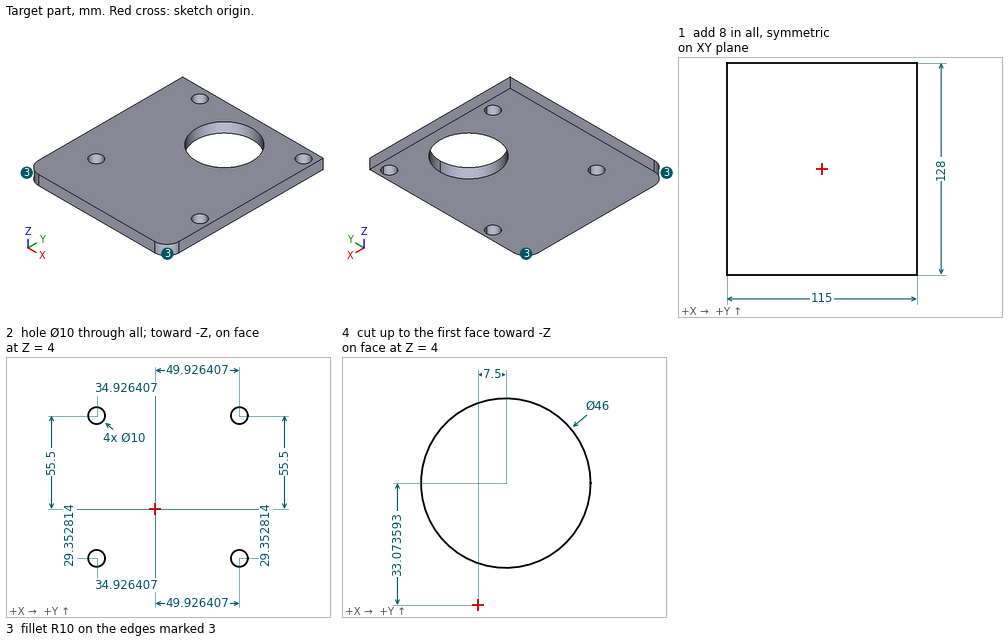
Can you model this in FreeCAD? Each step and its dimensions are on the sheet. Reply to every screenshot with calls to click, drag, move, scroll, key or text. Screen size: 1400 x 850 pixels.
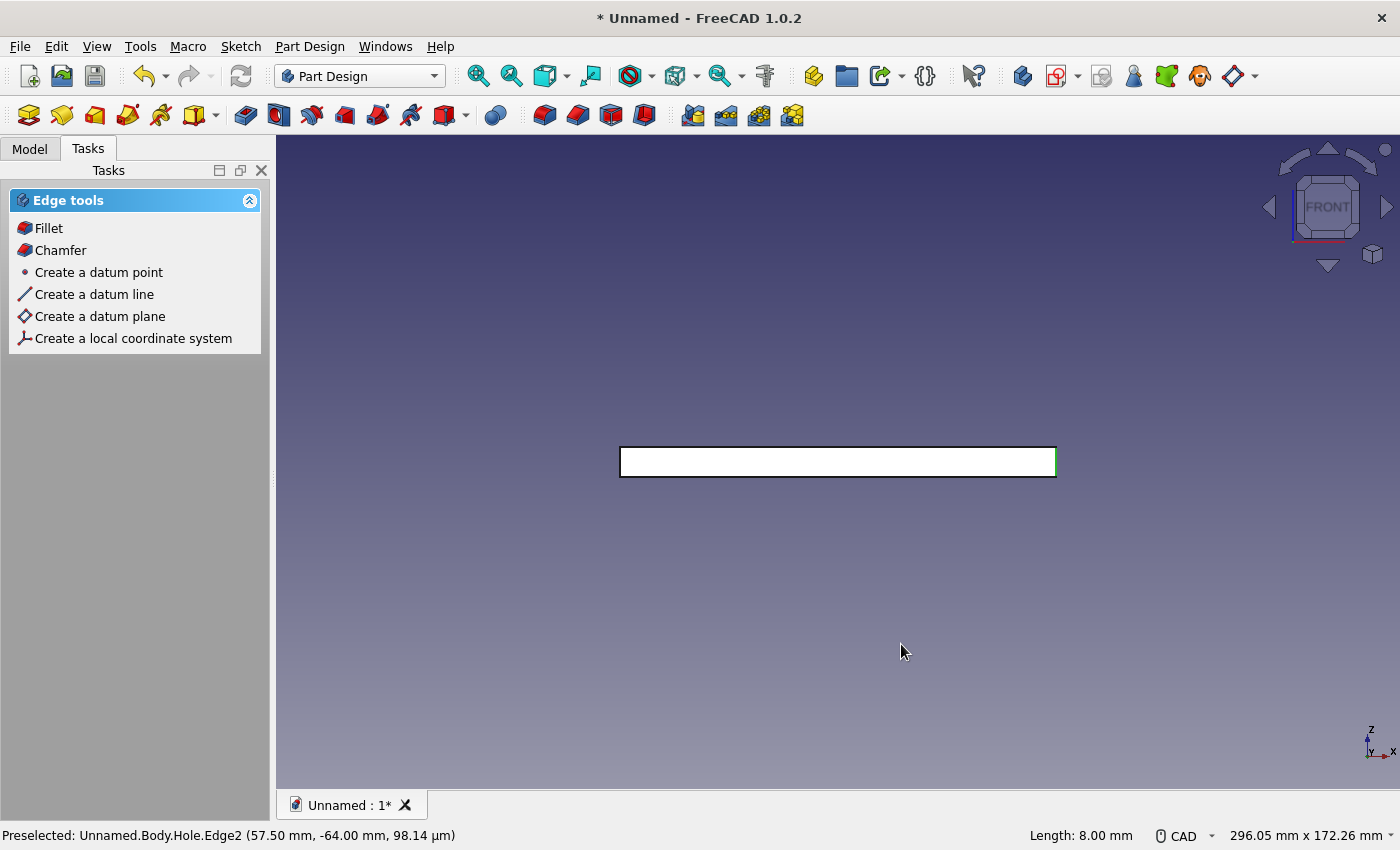
click(479, 76)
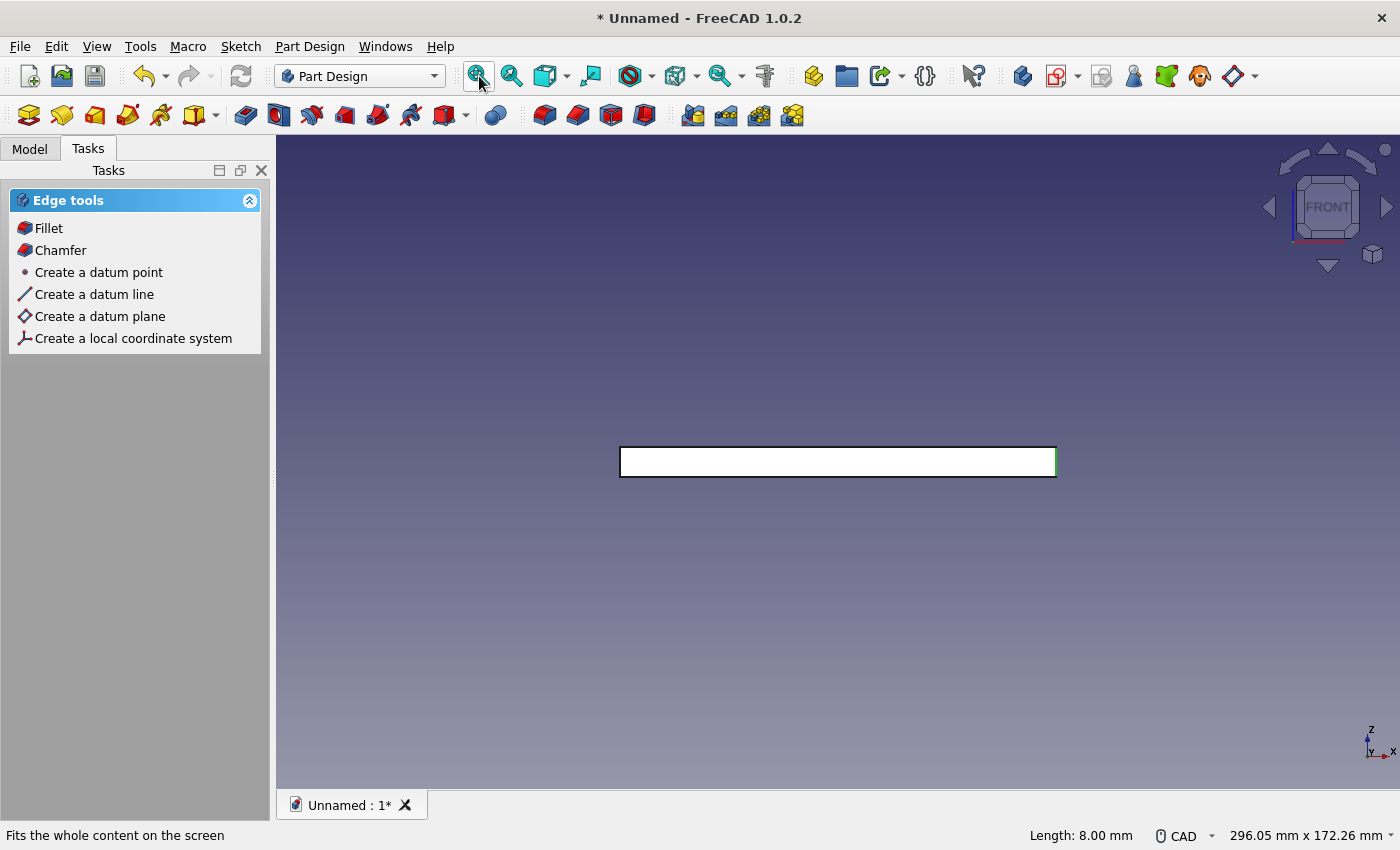
click(620, 461, ctrl)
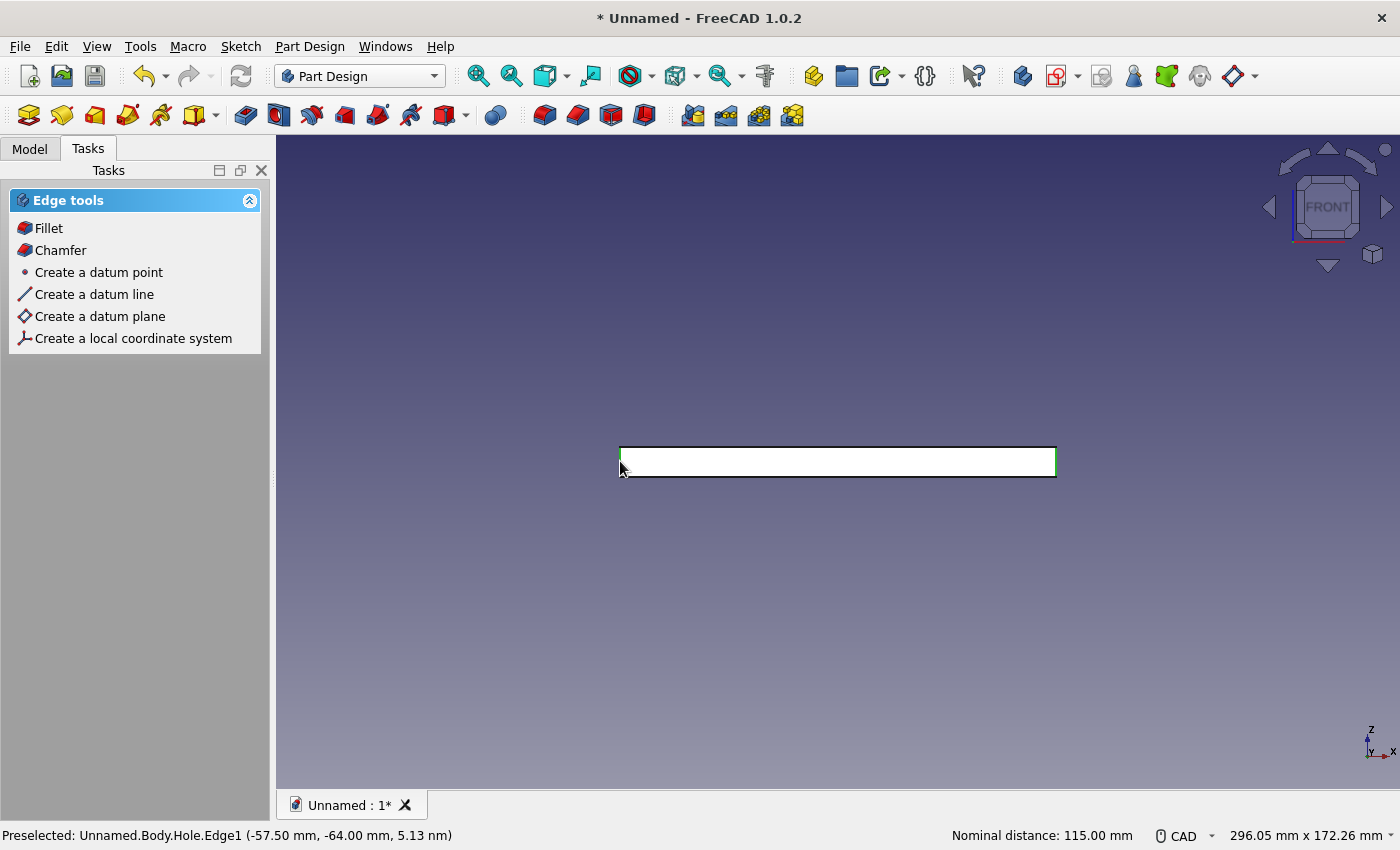
click(545, 116)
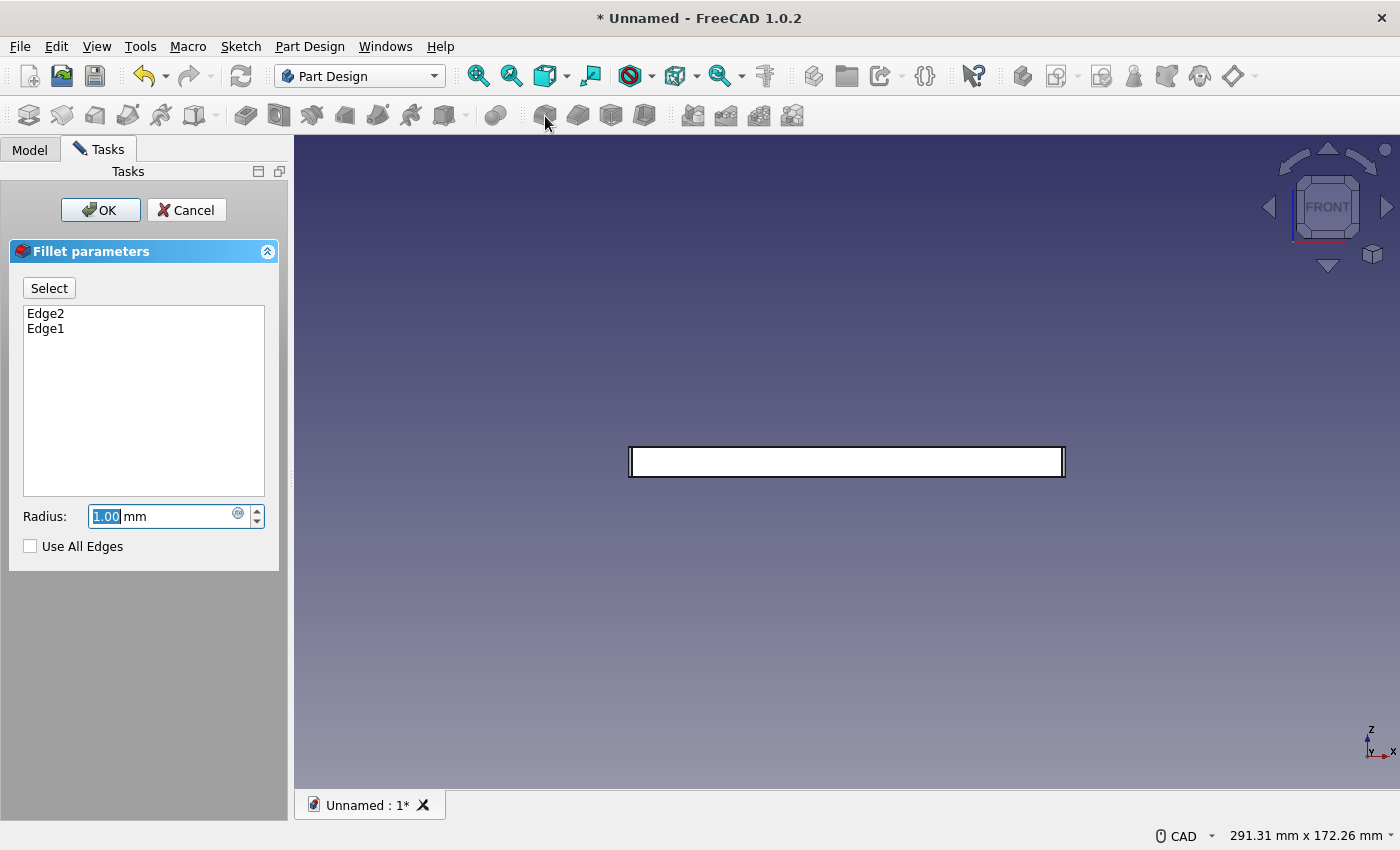
text(10)
key(Tab)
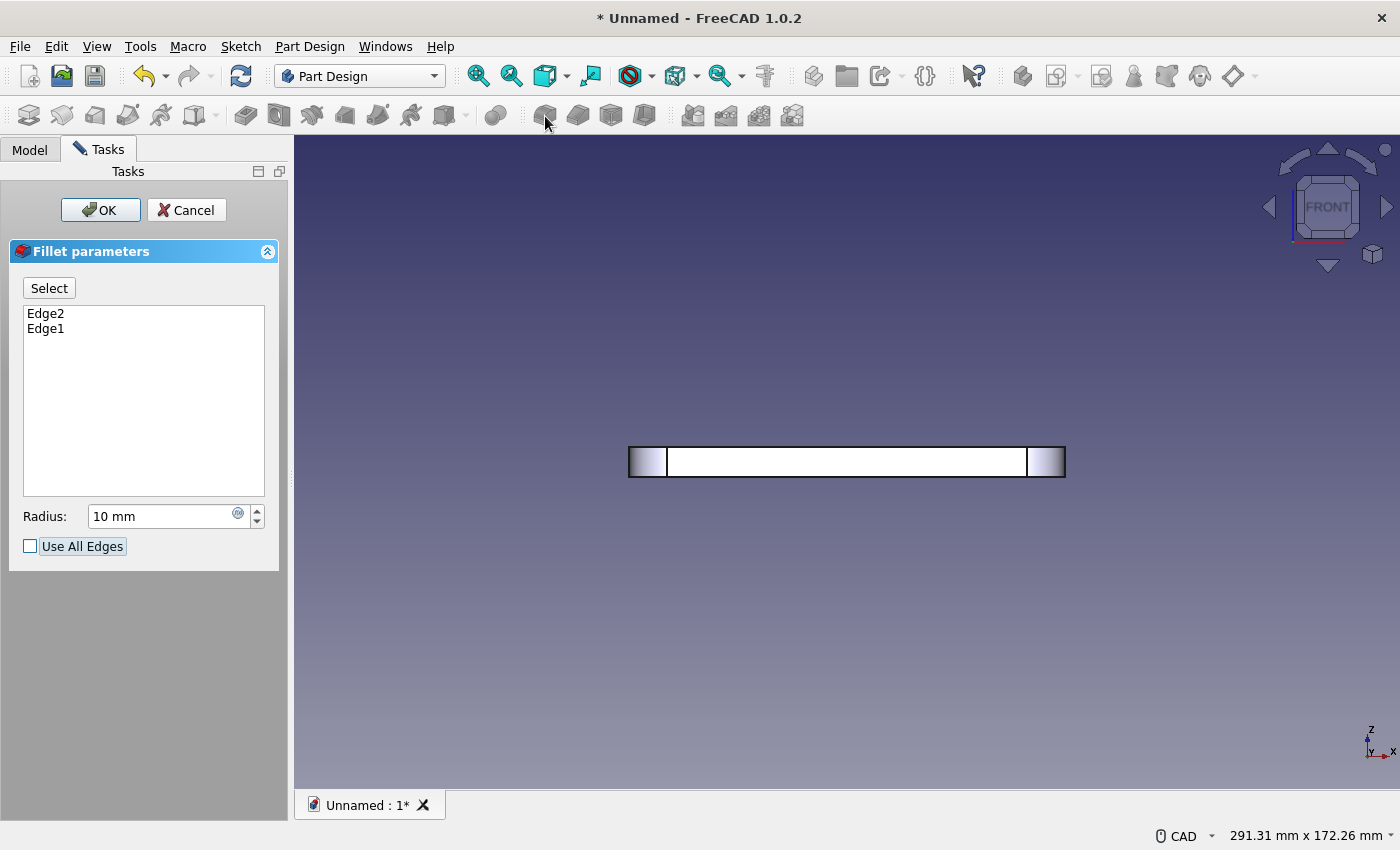
click(101, 210)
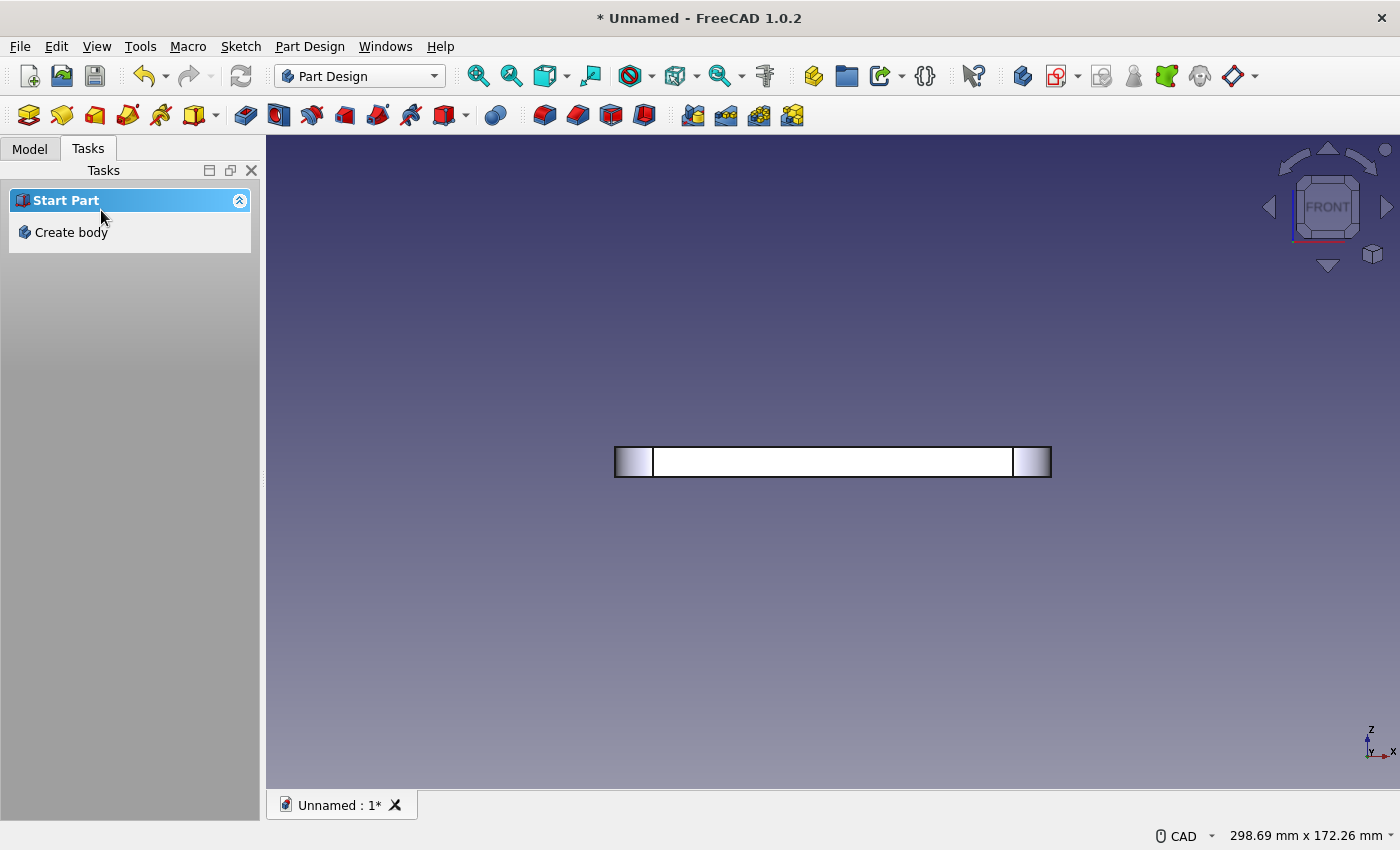
click(479, 76)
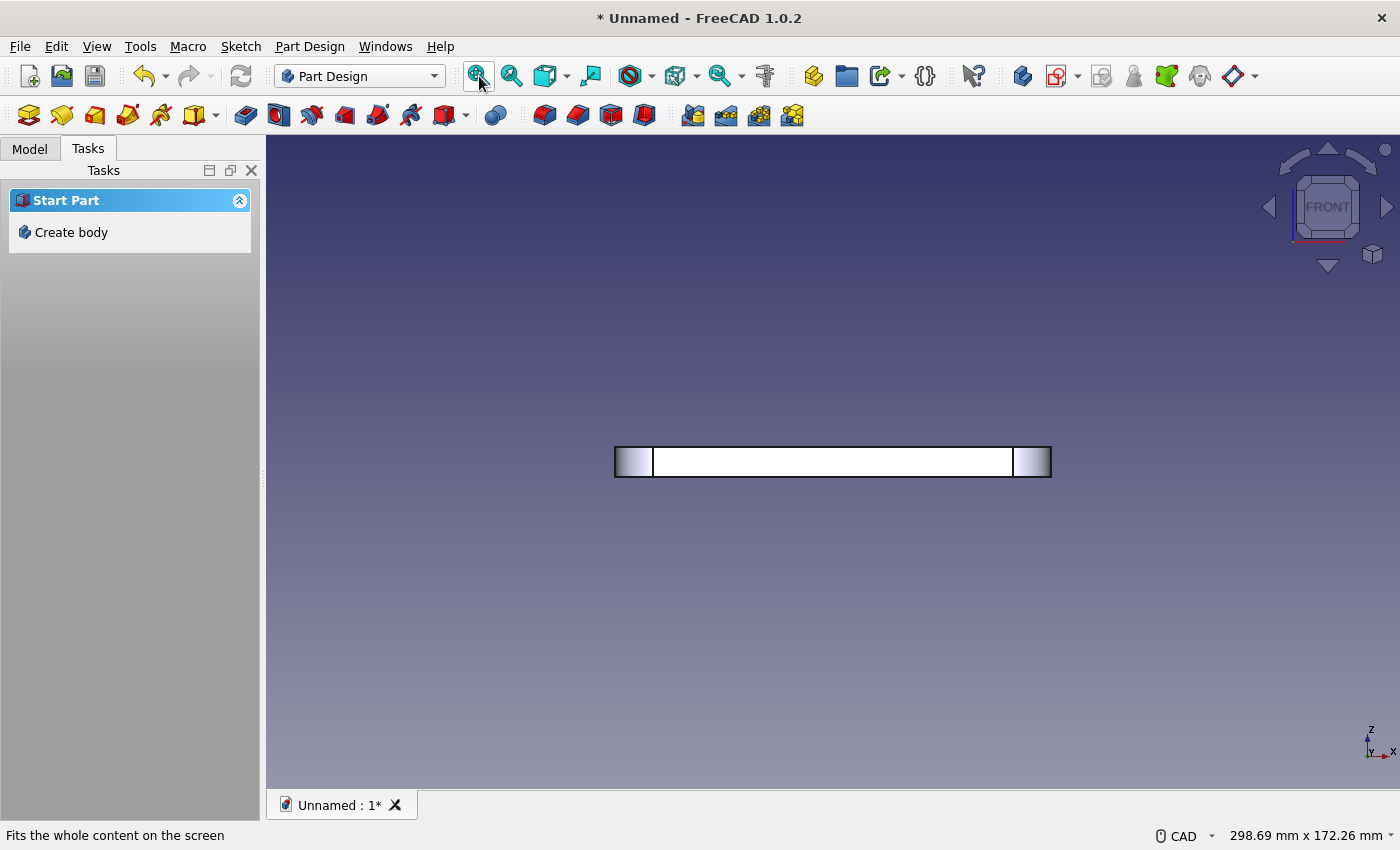
key(0)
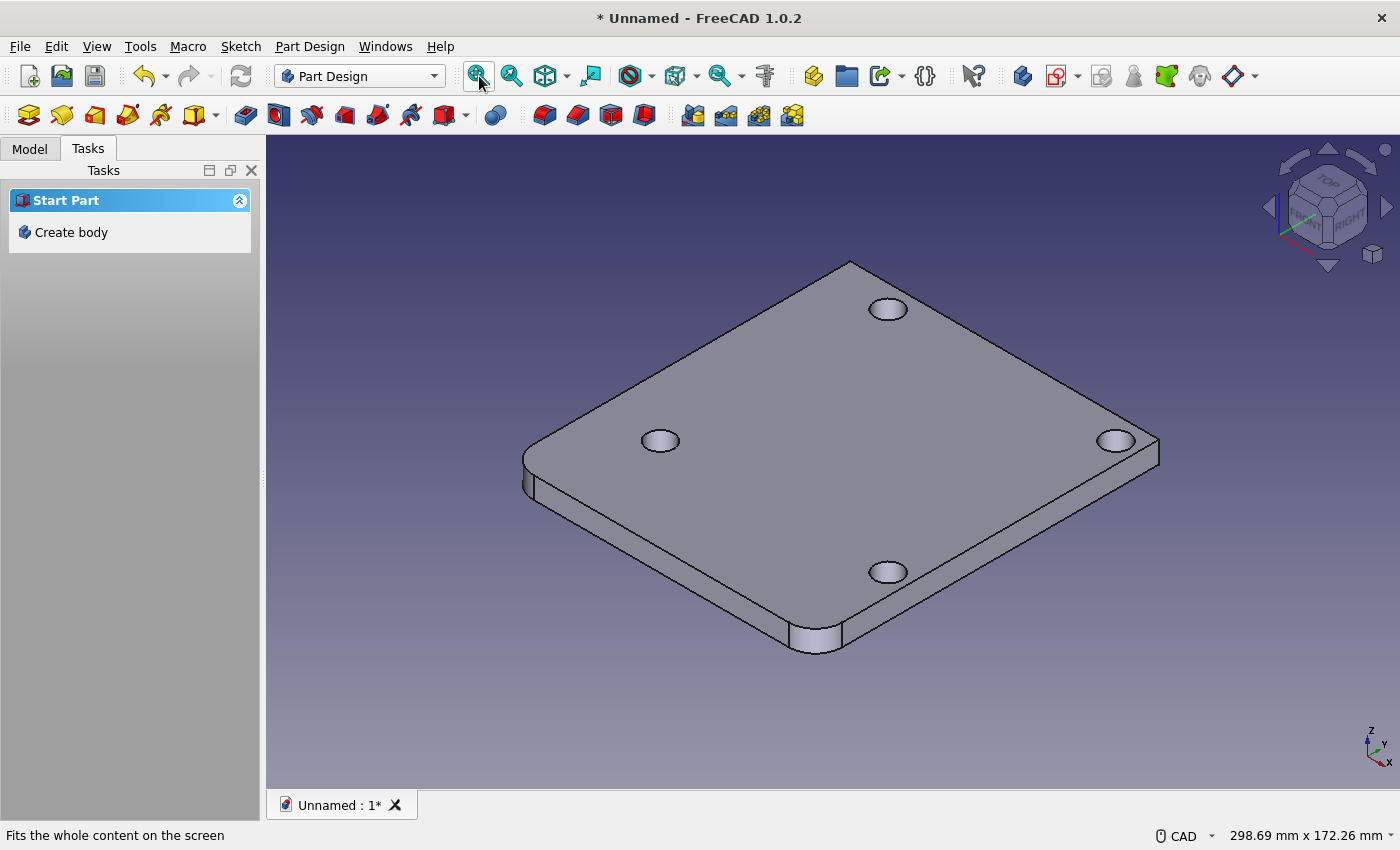
click(882, 420)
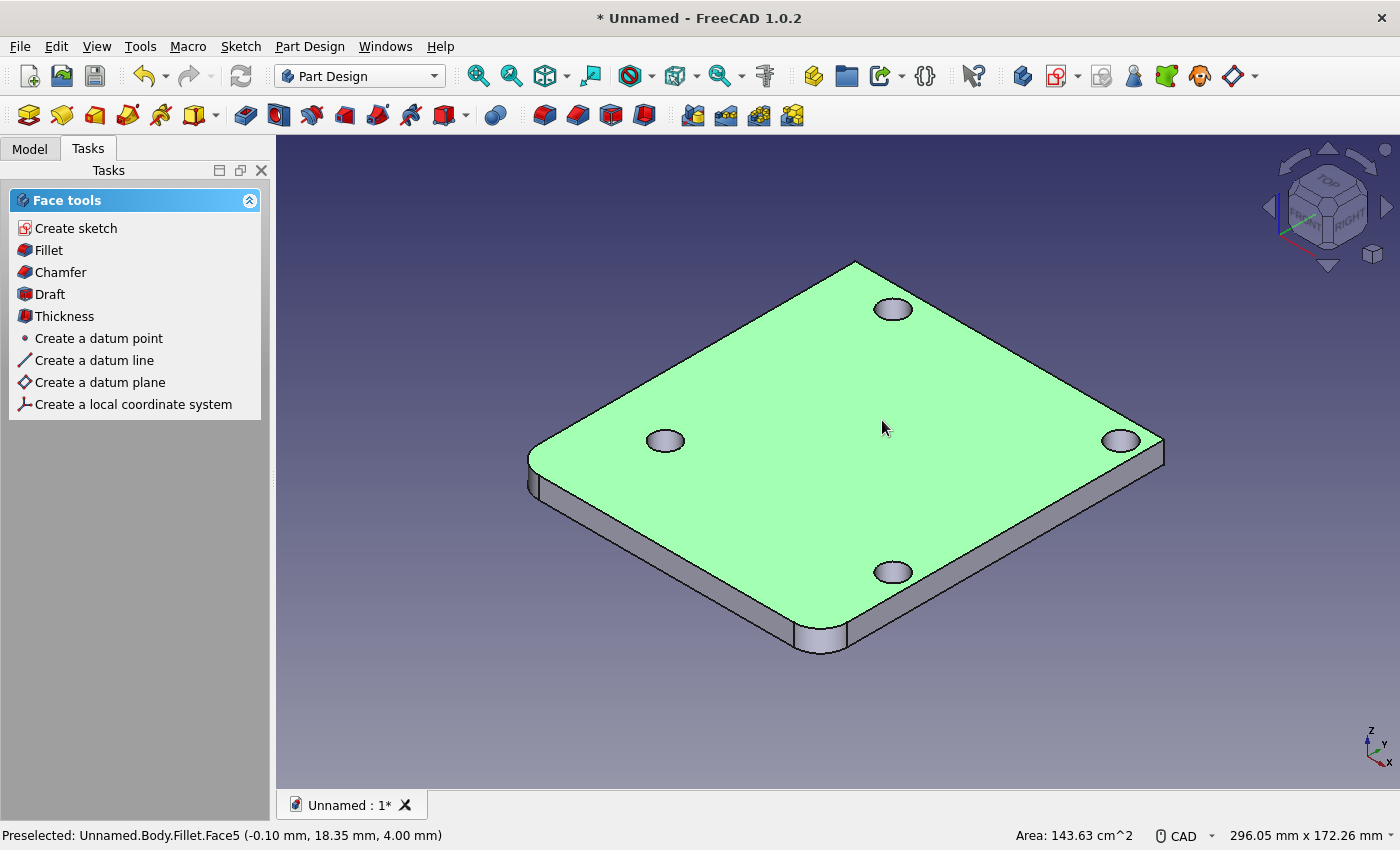
click(1056, 76)